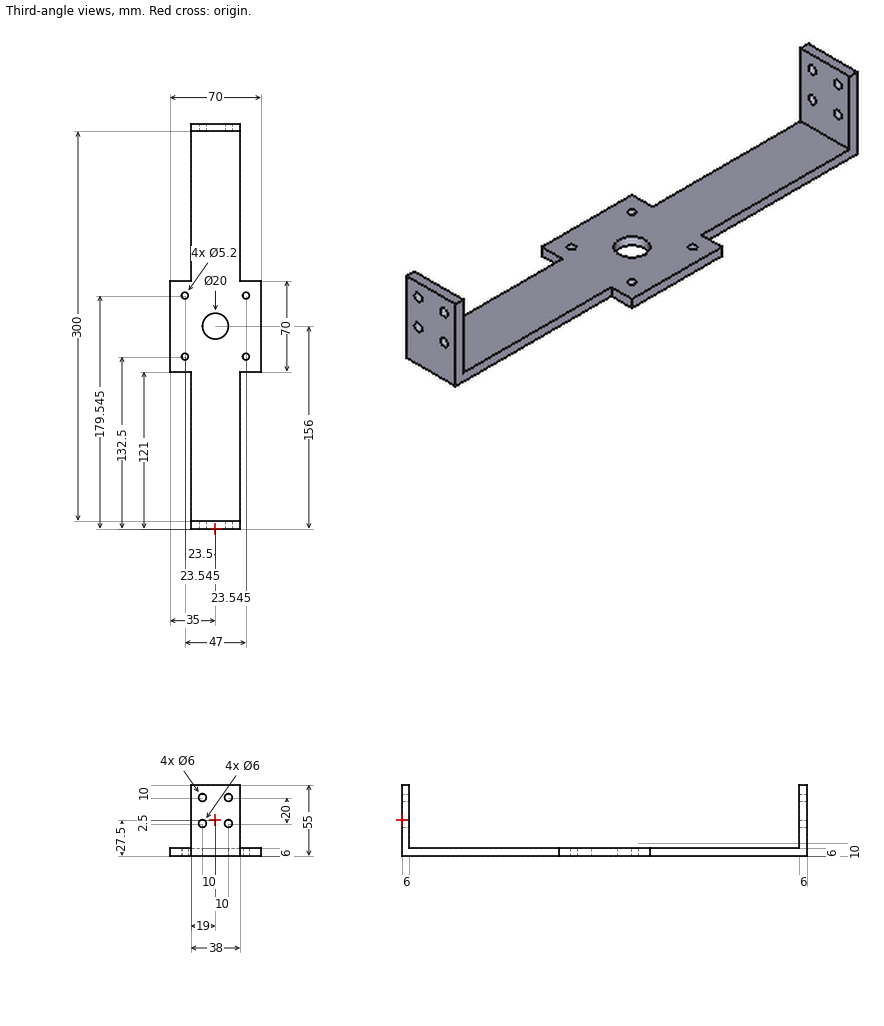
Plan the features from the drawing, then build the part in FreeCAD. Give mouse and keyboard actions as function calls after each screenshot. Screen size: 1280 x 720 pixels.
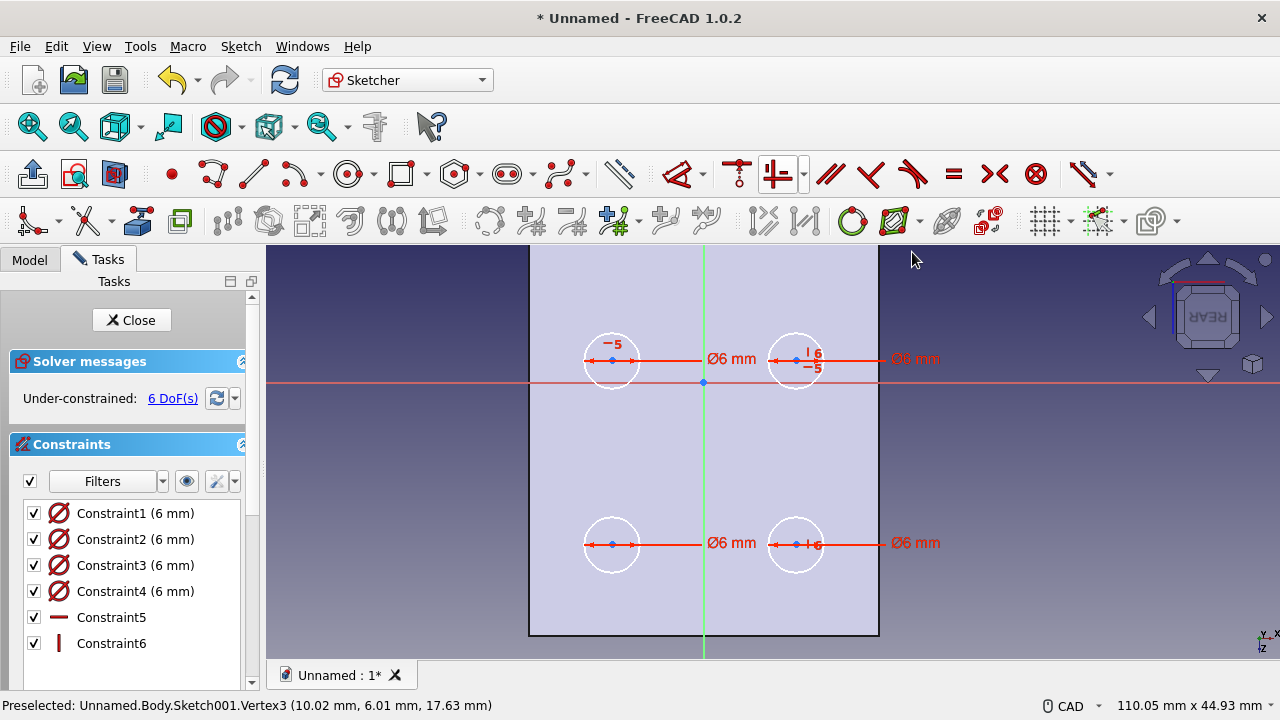
click(612, 361)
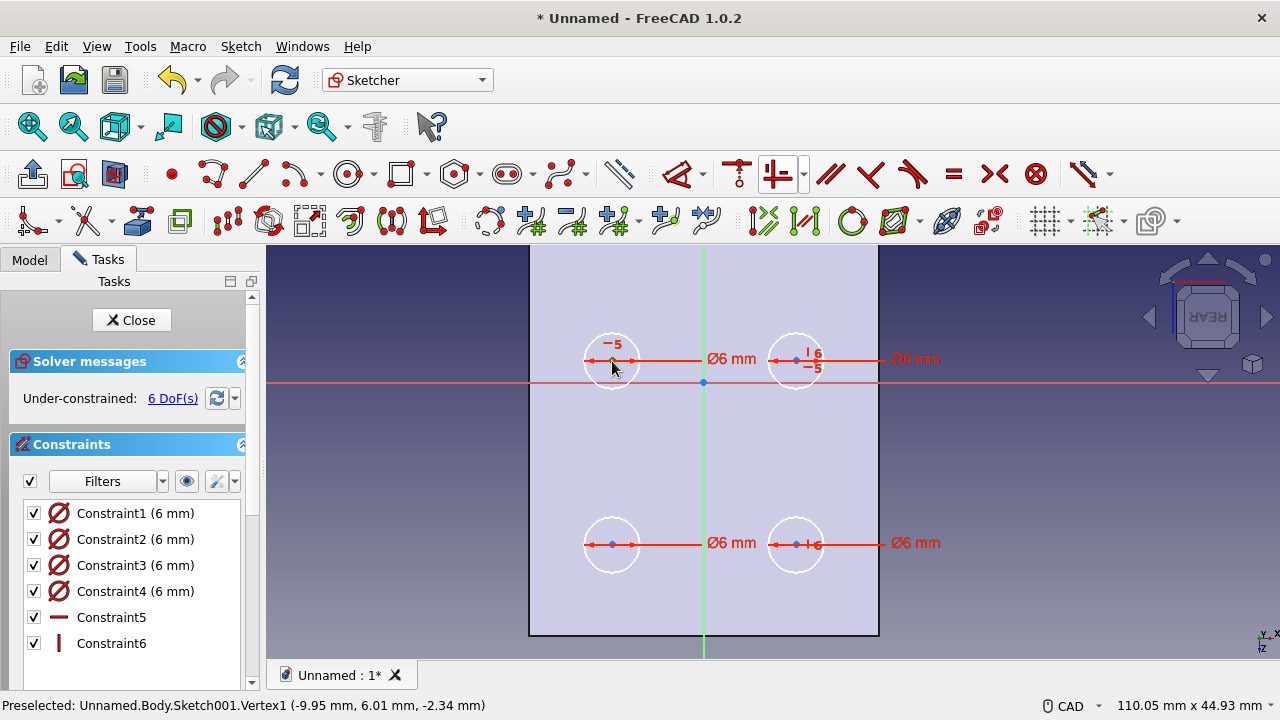
click(612, 545)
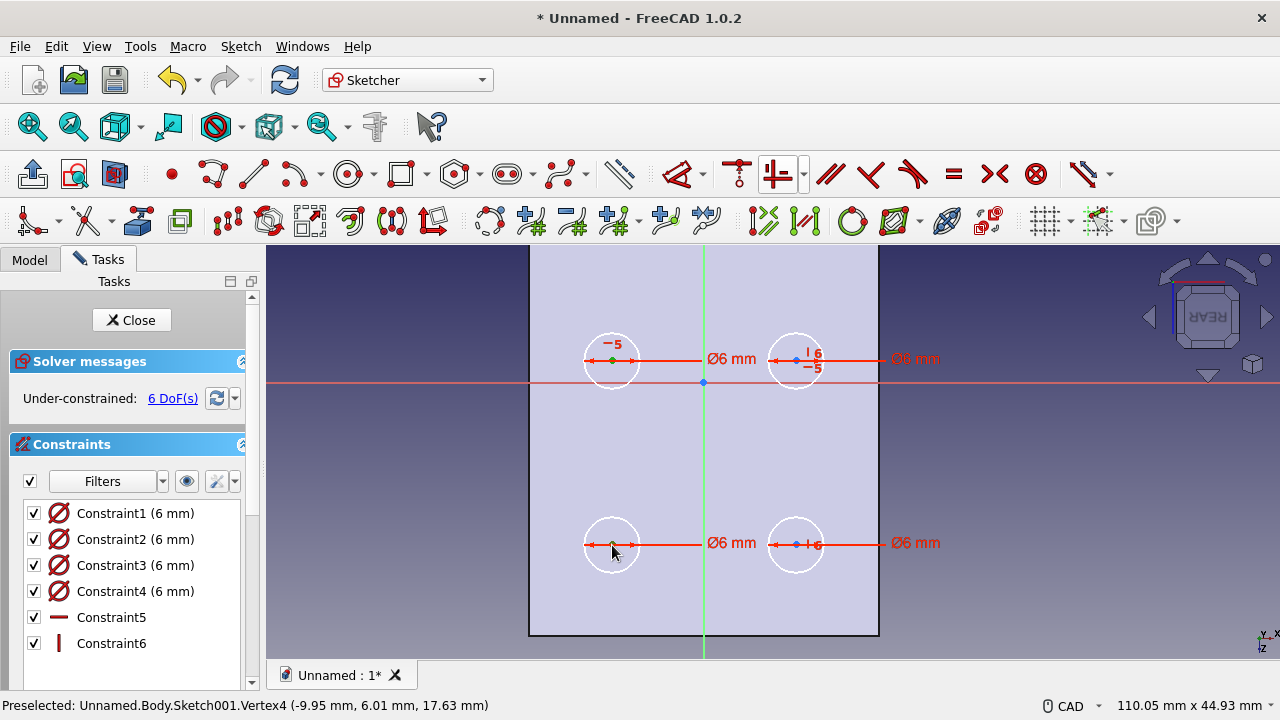
click(804, 174)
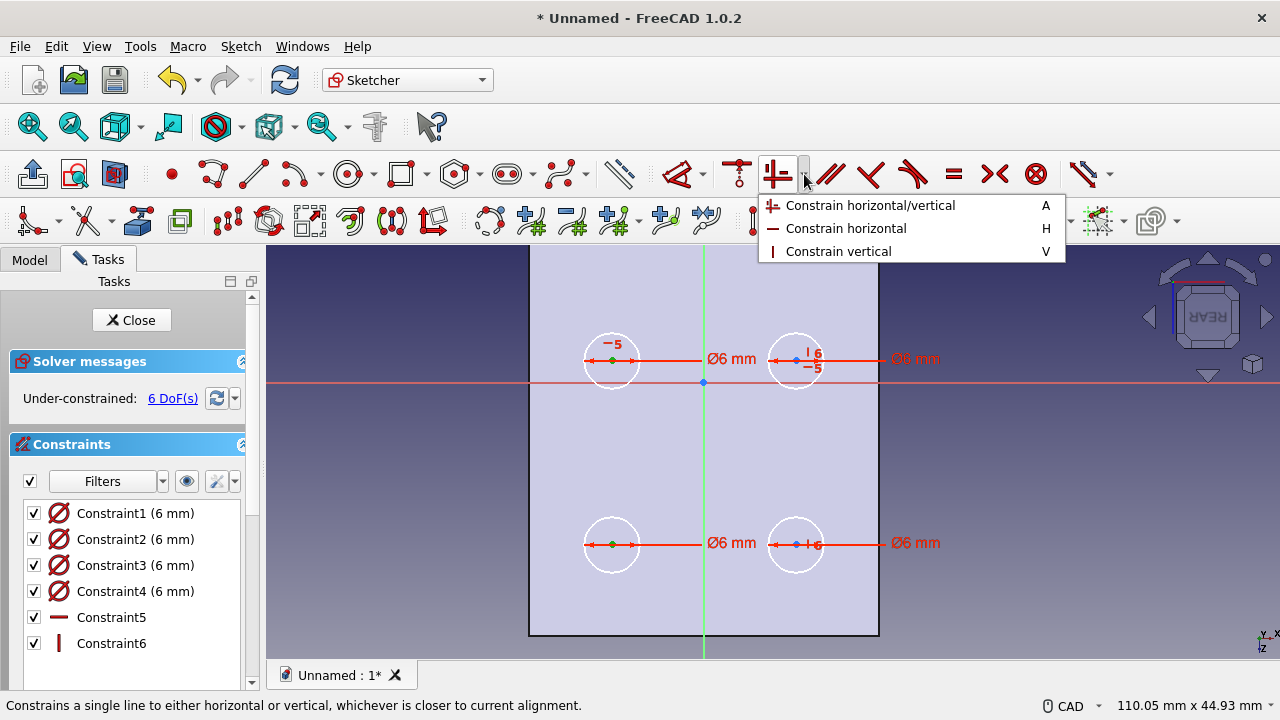
click(912, 252)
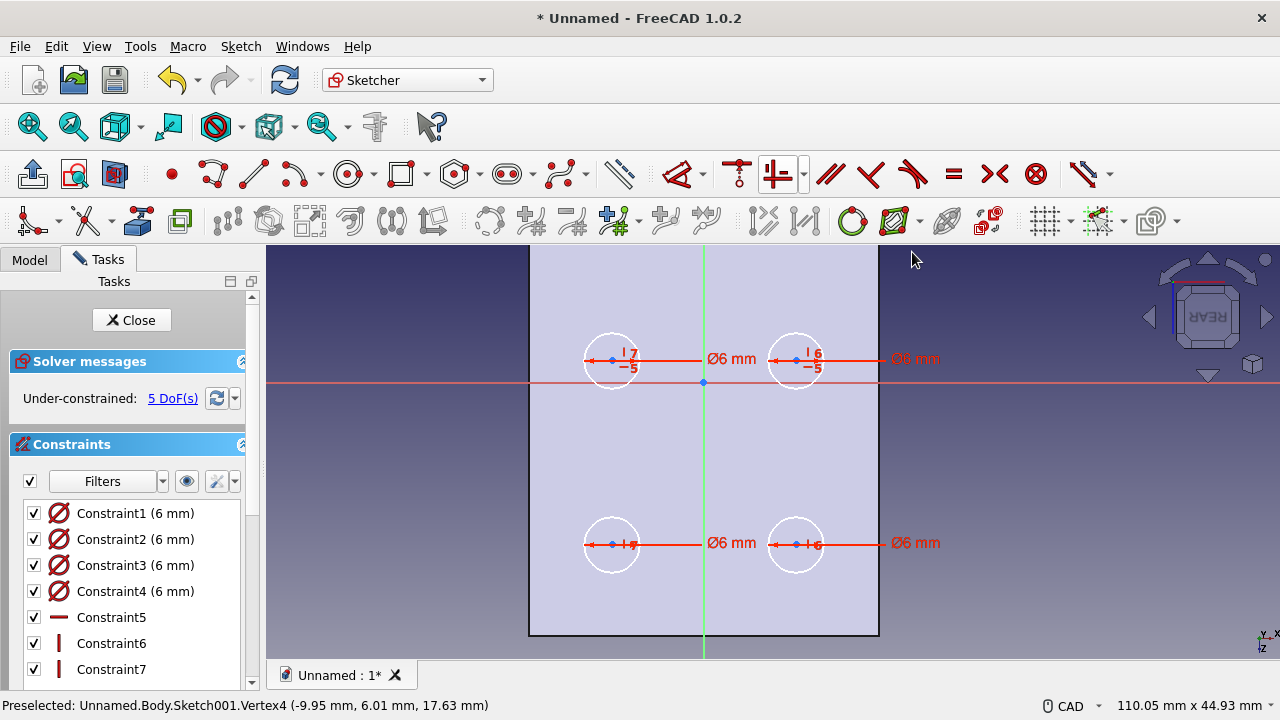
click(796, 545)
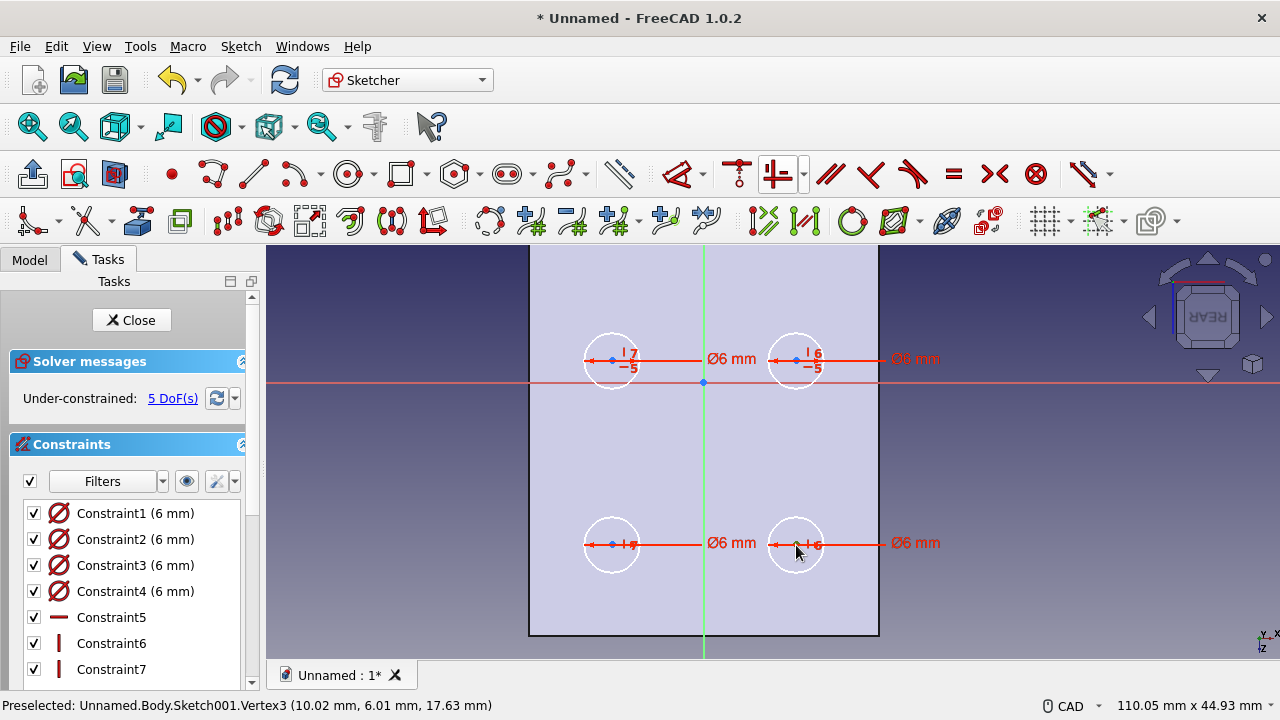
click(612, 545)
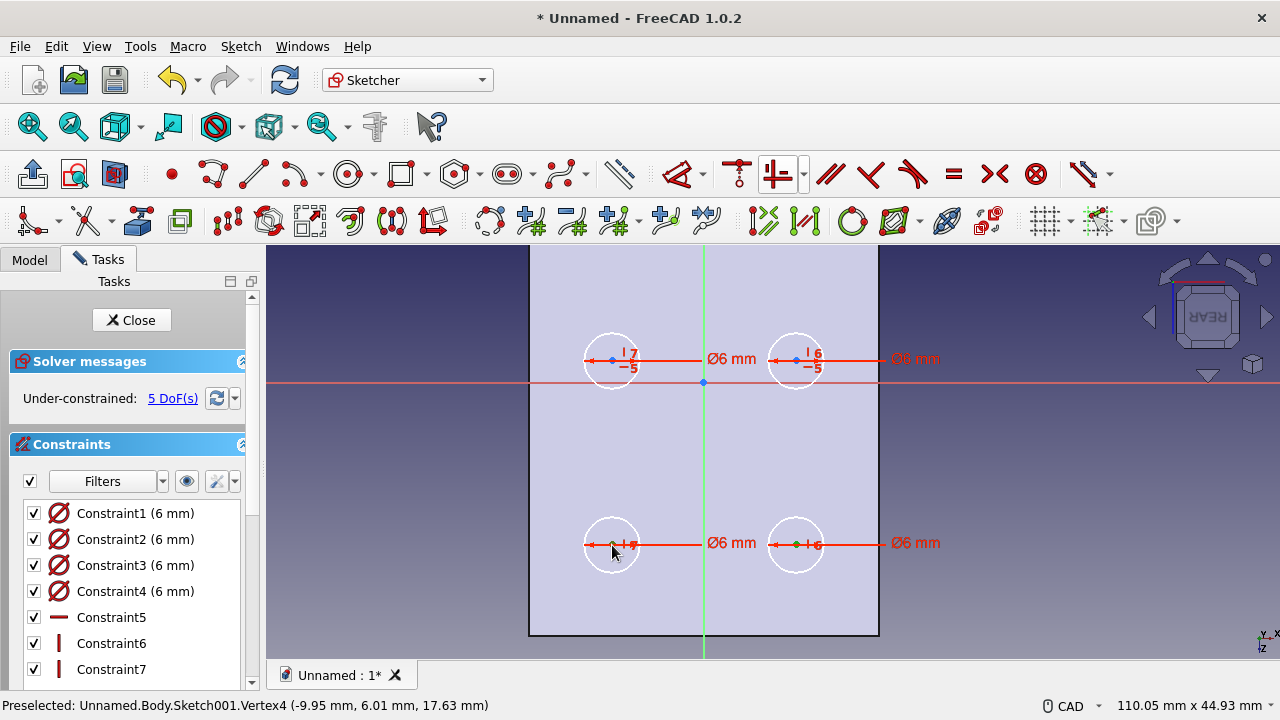
click(804, 174)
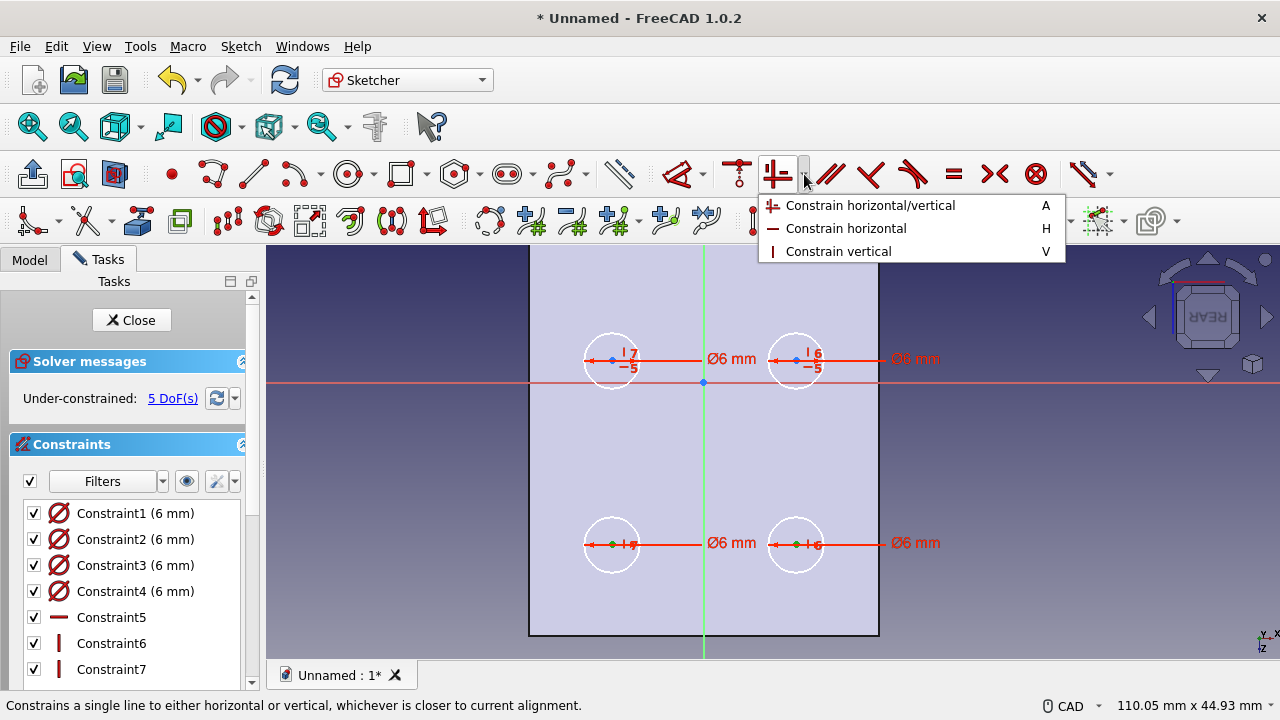
click(912, 228)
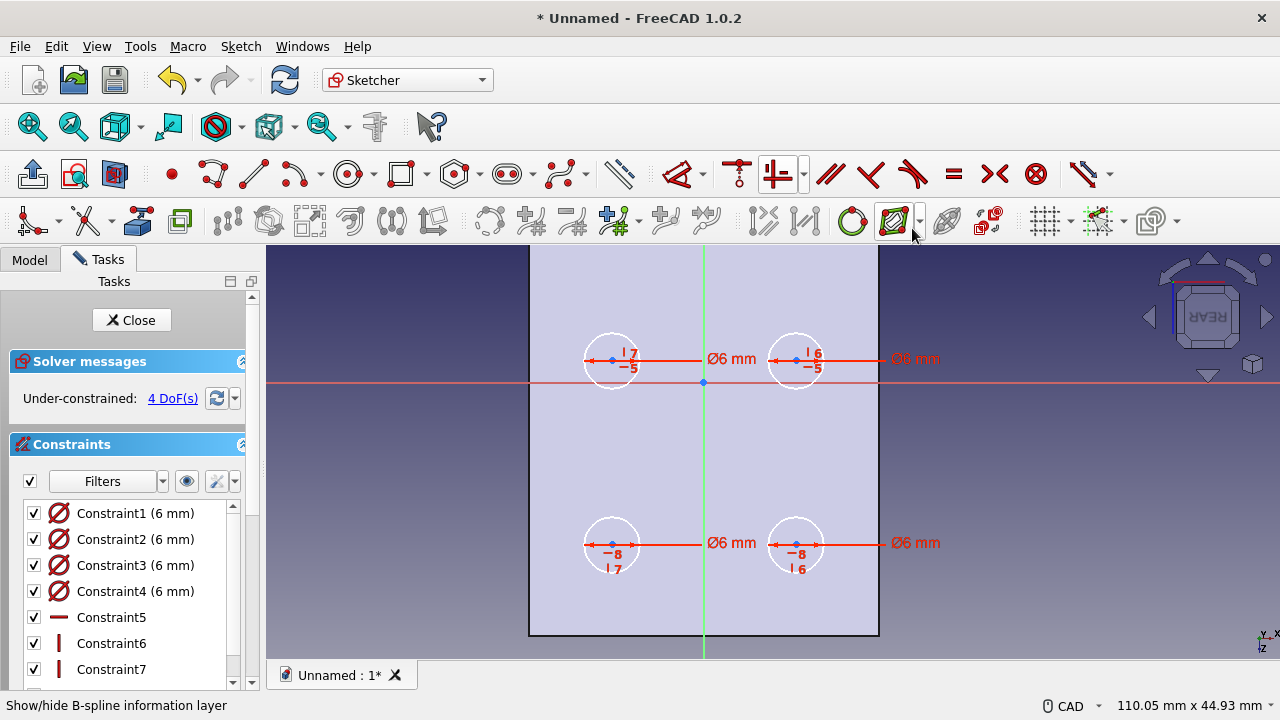
click(676, 174)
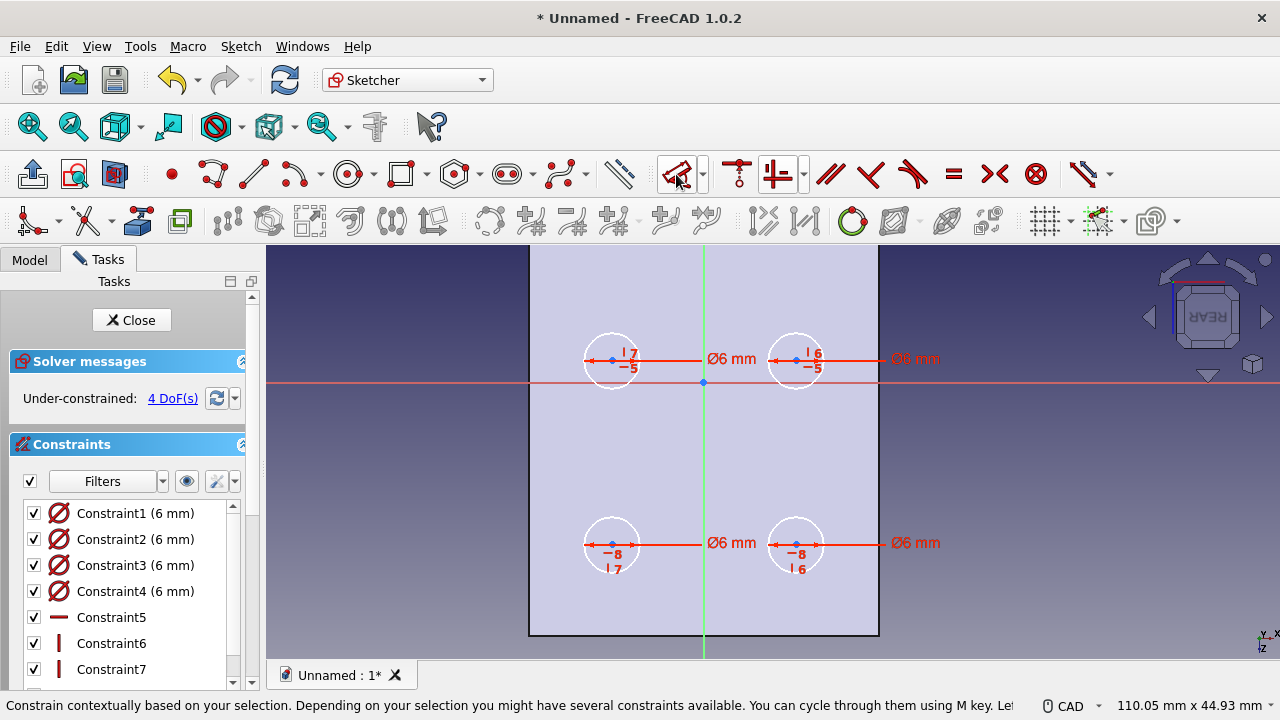
click(612, 361)
click(658, 327)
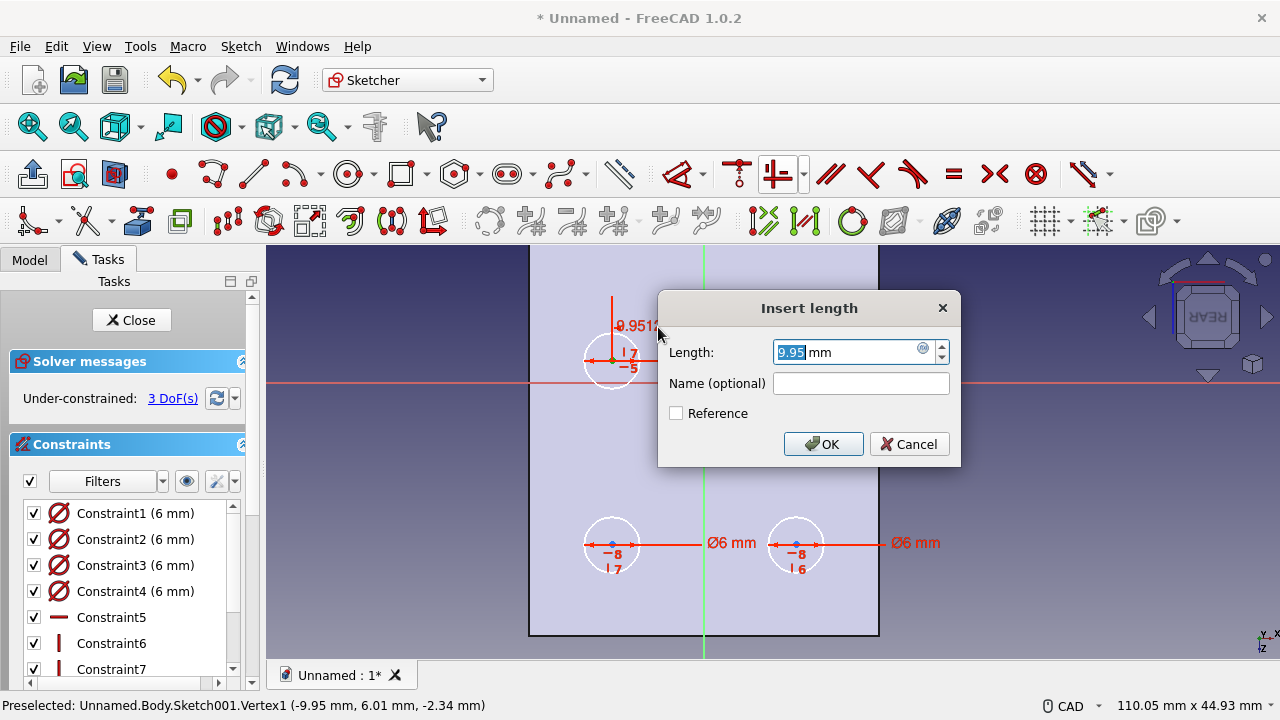
text(10)
key(Return)